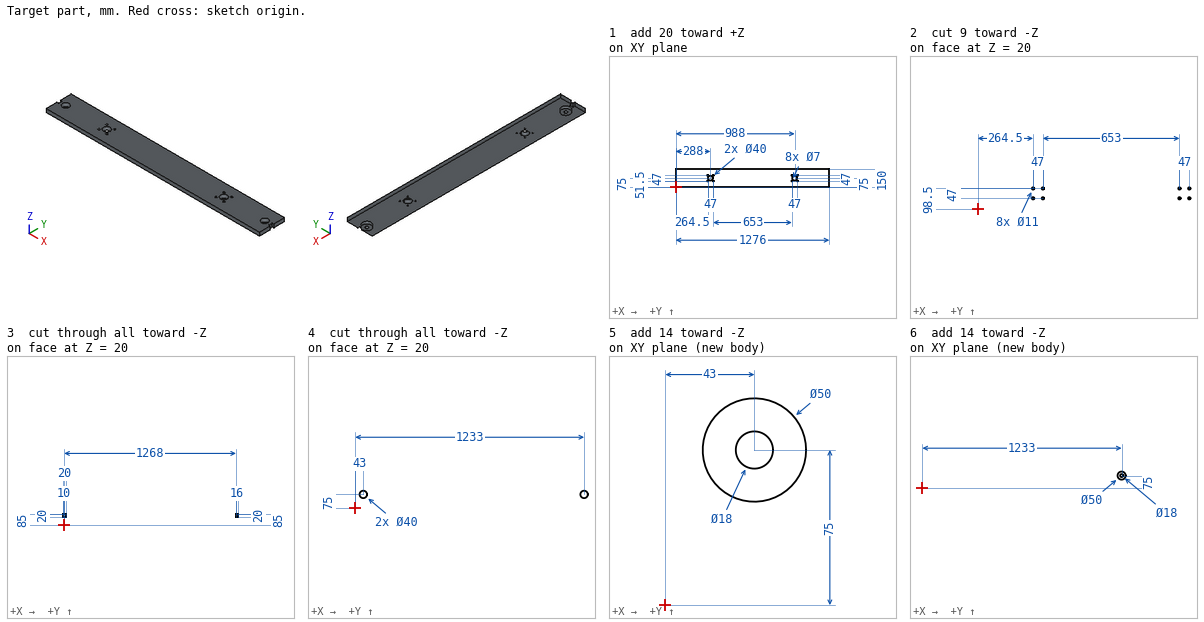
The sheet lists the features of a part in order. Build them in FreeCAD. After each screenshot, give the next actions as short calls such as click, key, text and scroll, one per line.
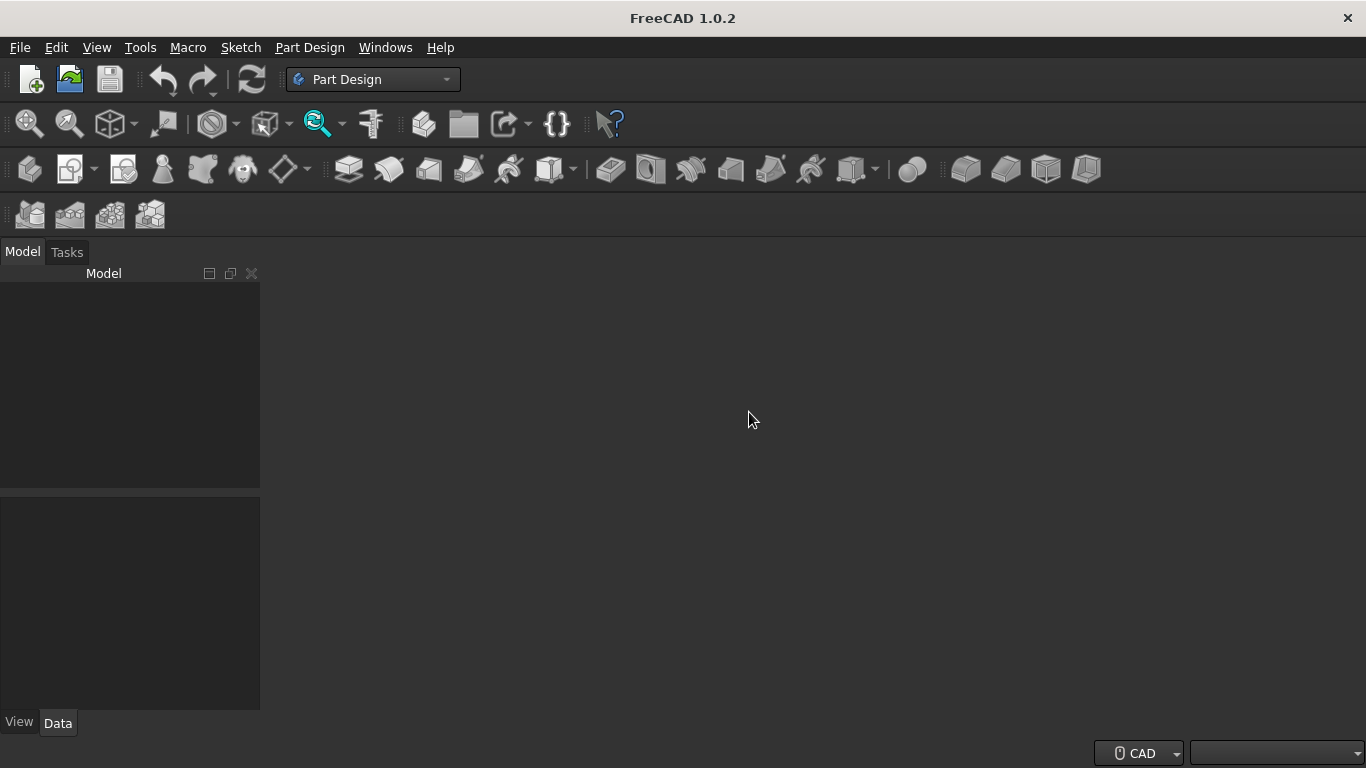
click(30, 80)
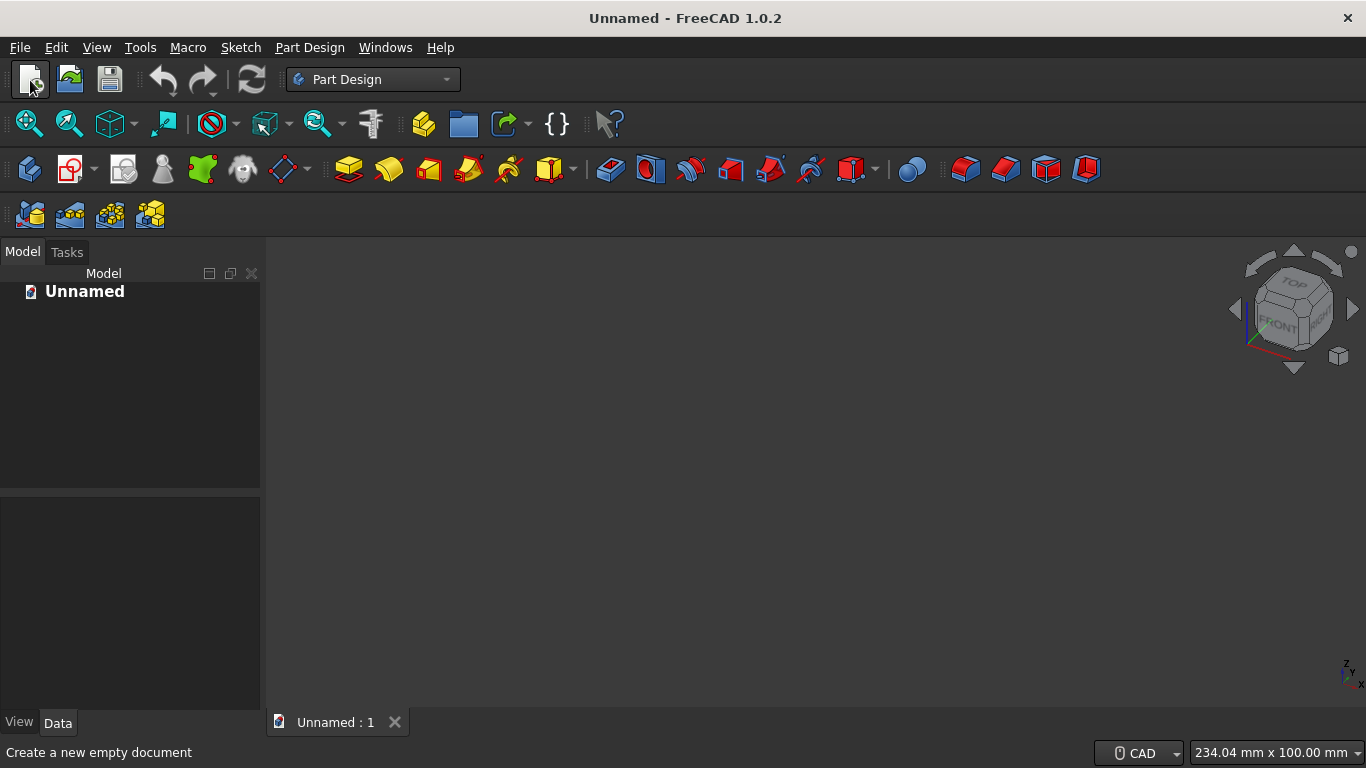
click(70, 170)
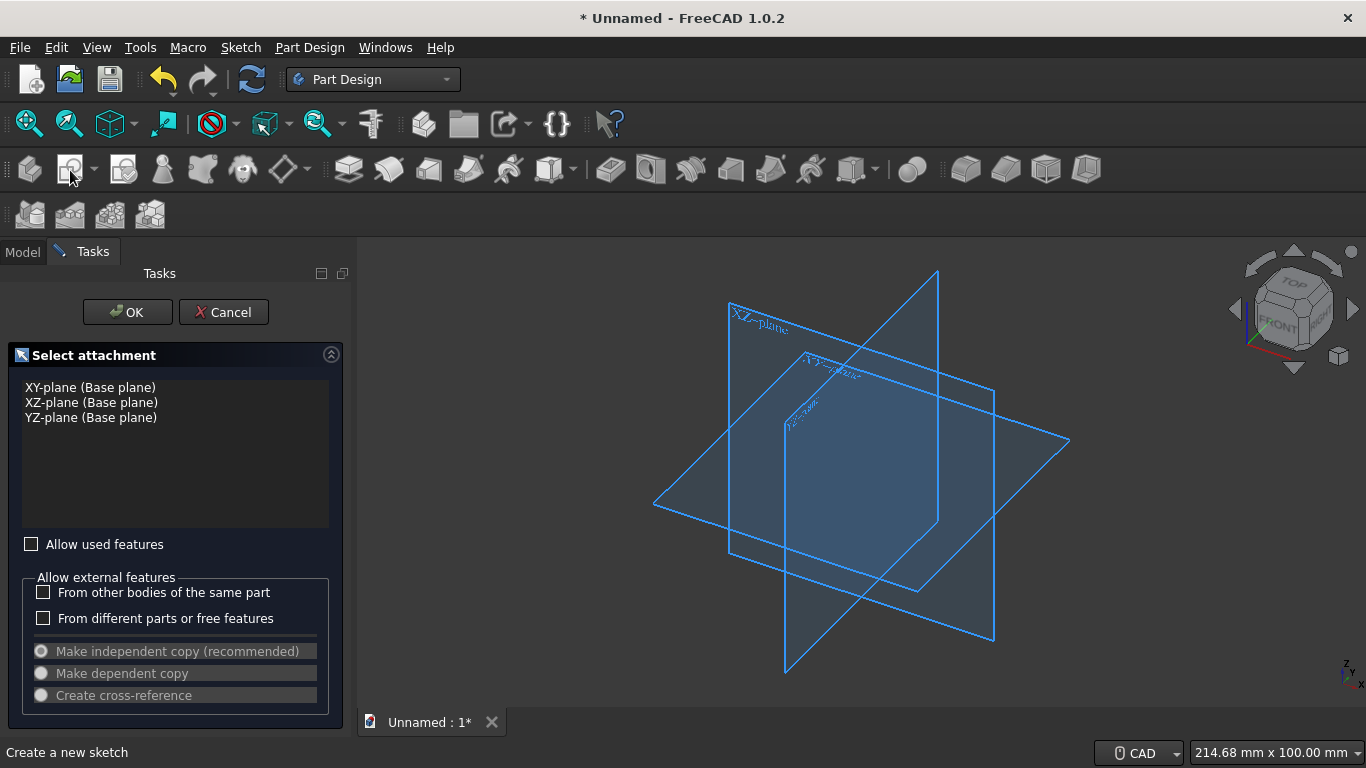
click(82, 388)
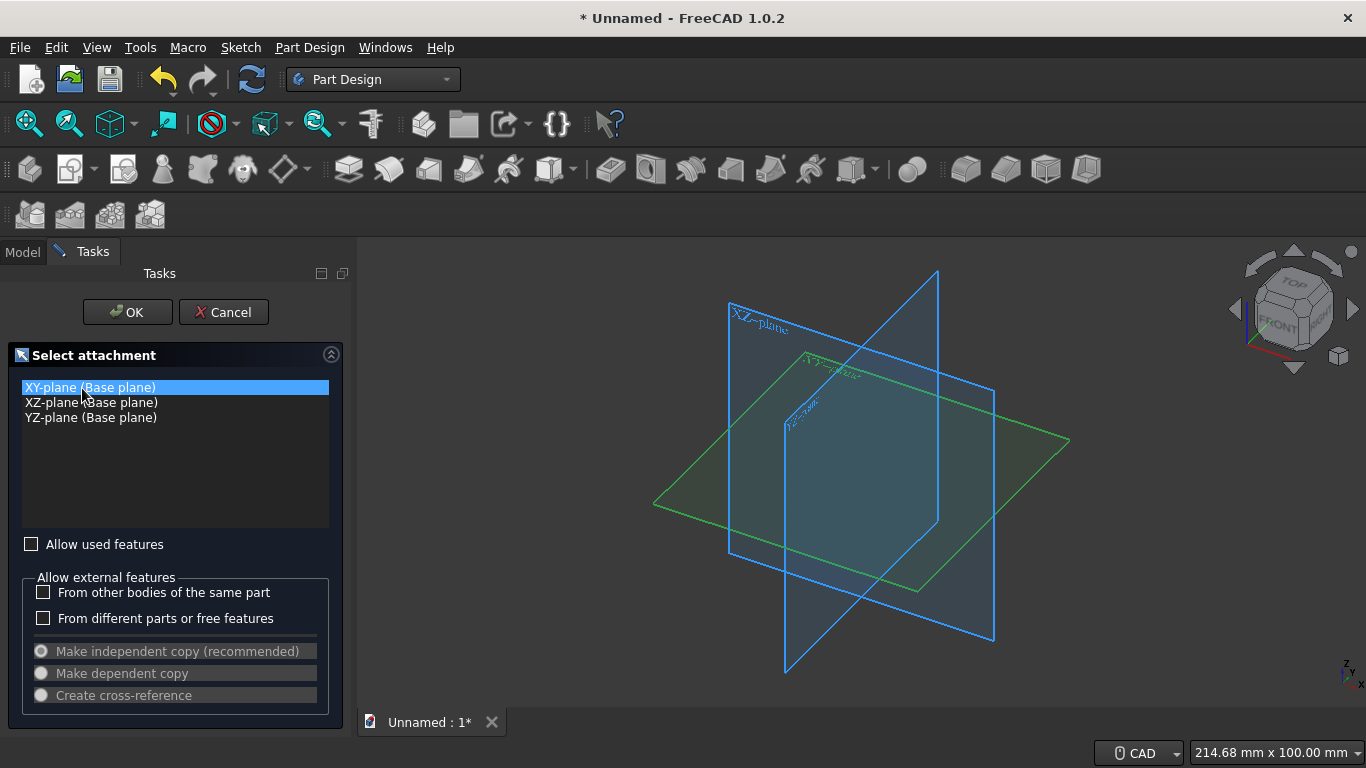
click(128, 312)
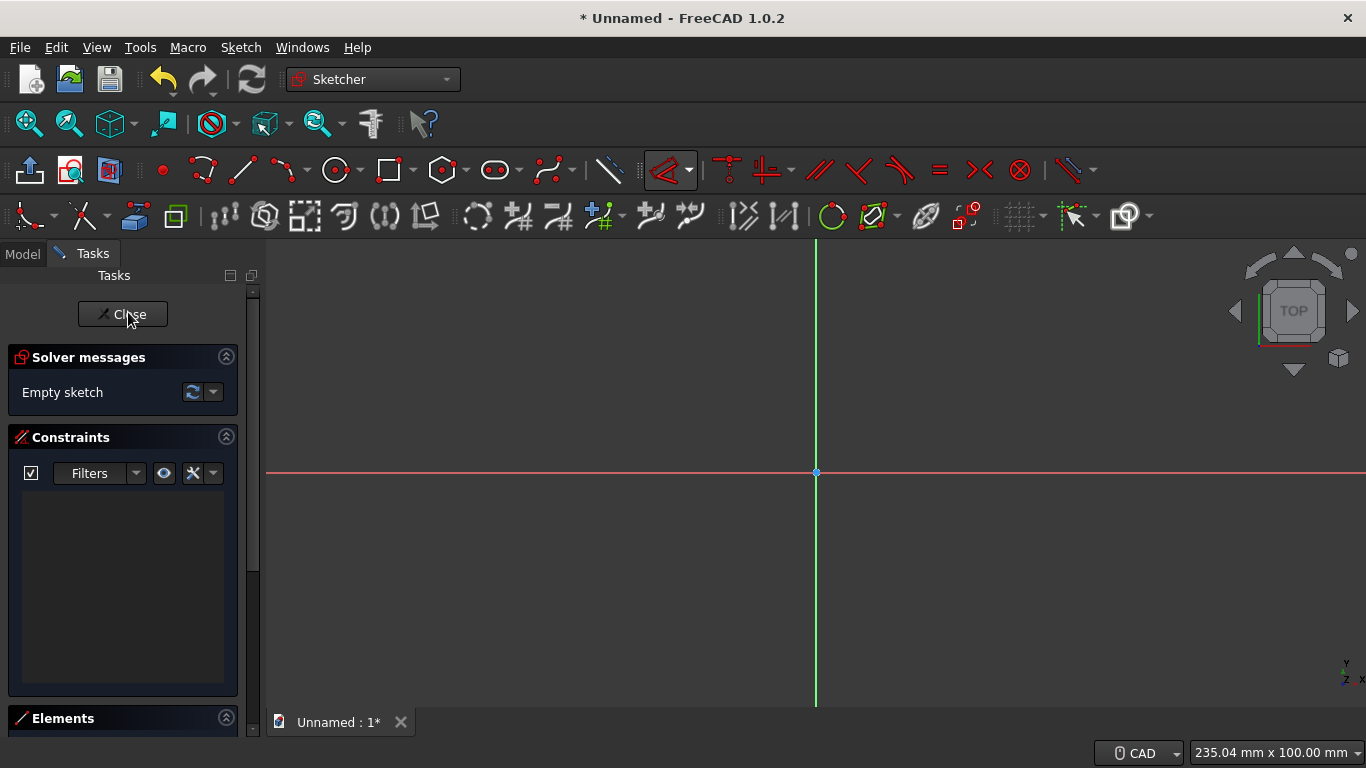
scroll(367, 517, down, 11)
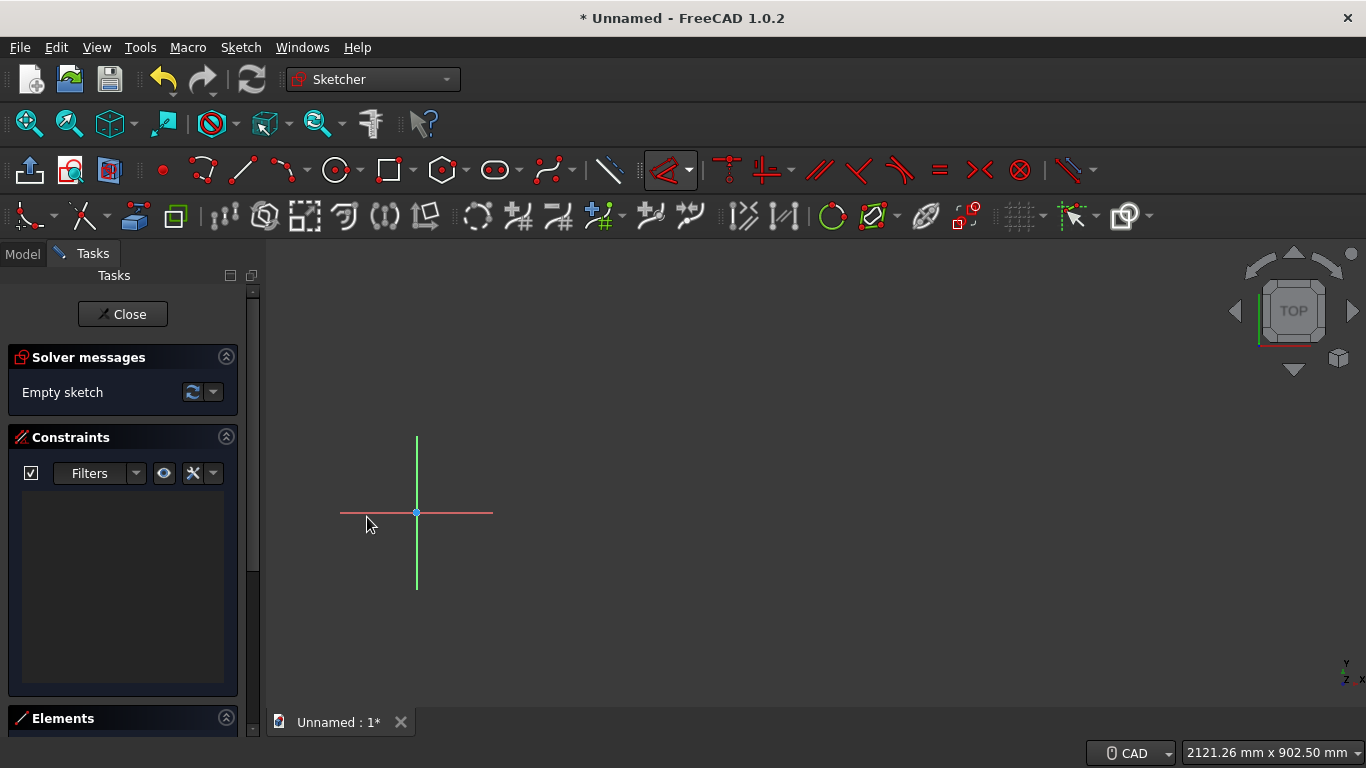
click(390, 170)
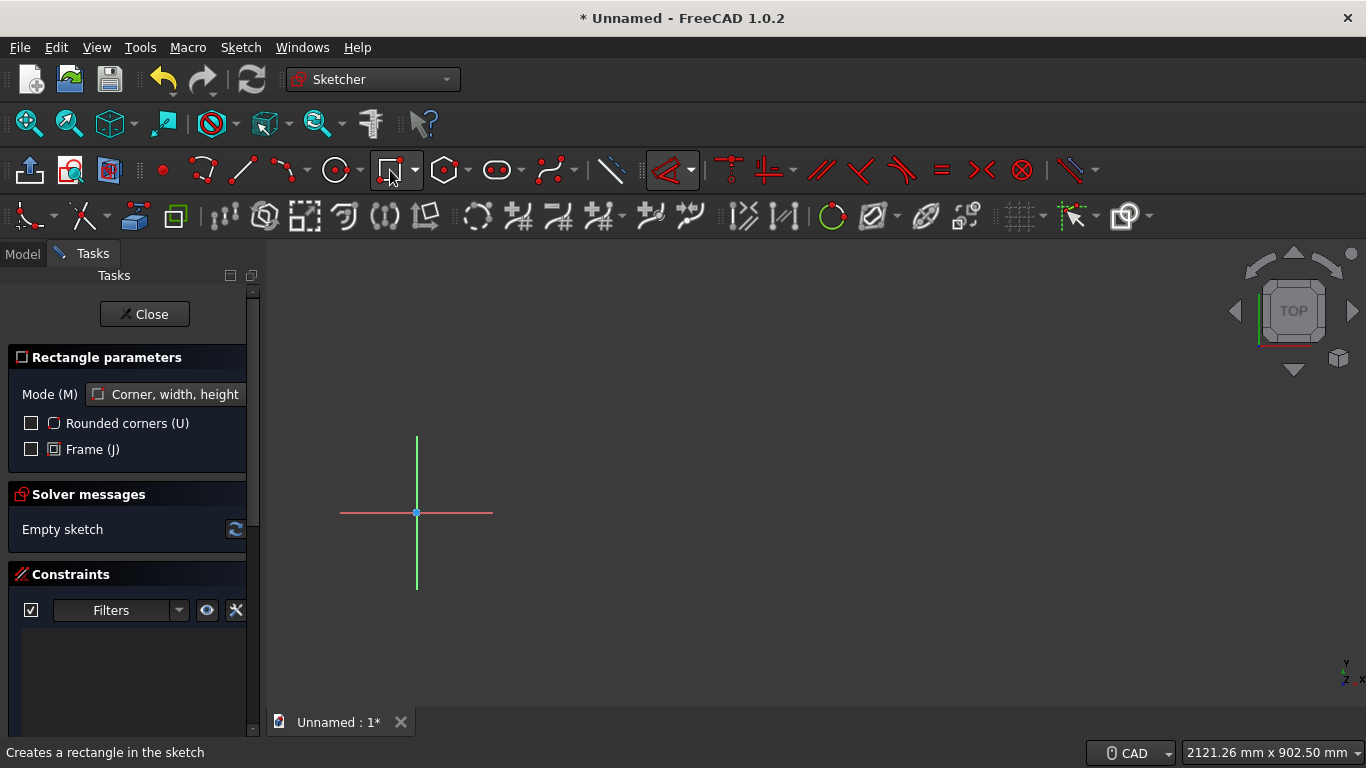
click(417, 513)
move(1079, 435)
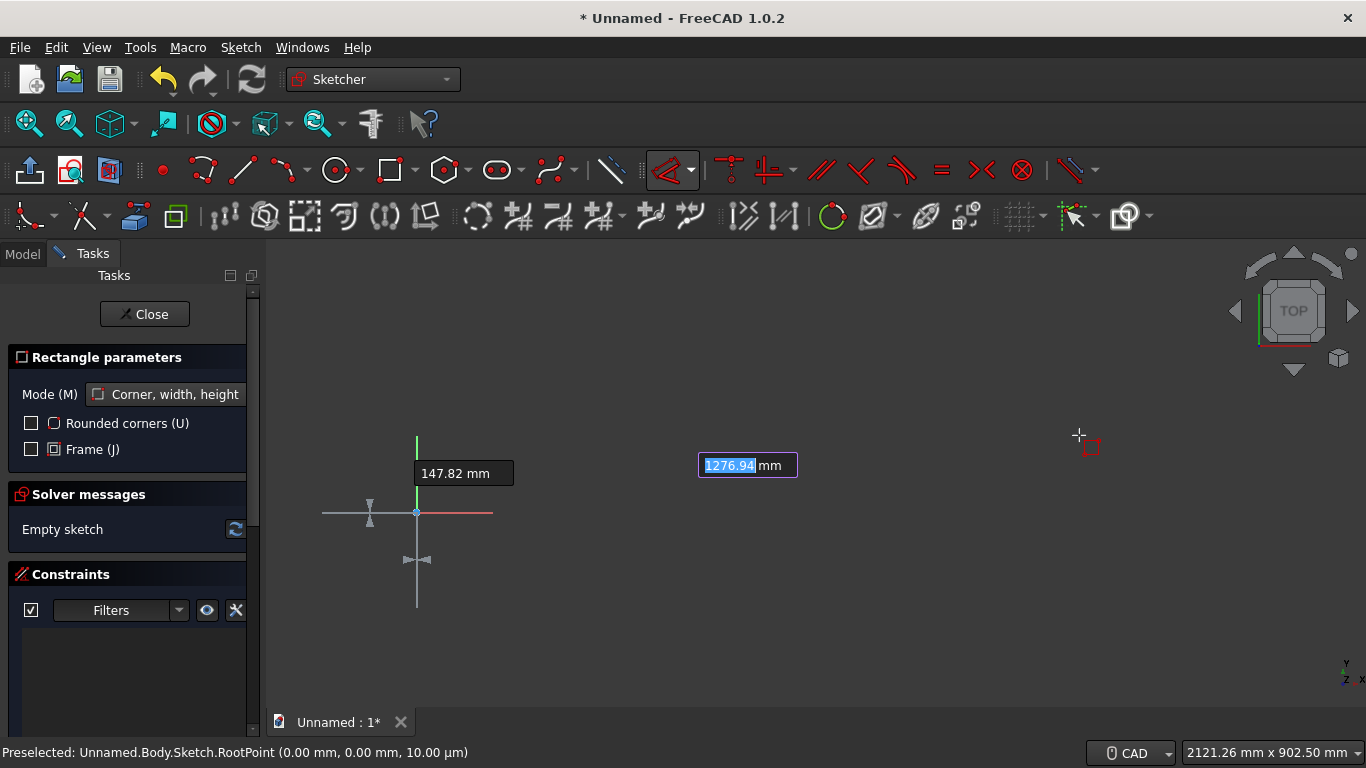
text(1276)
key(Tab)
text(150)
key(Return)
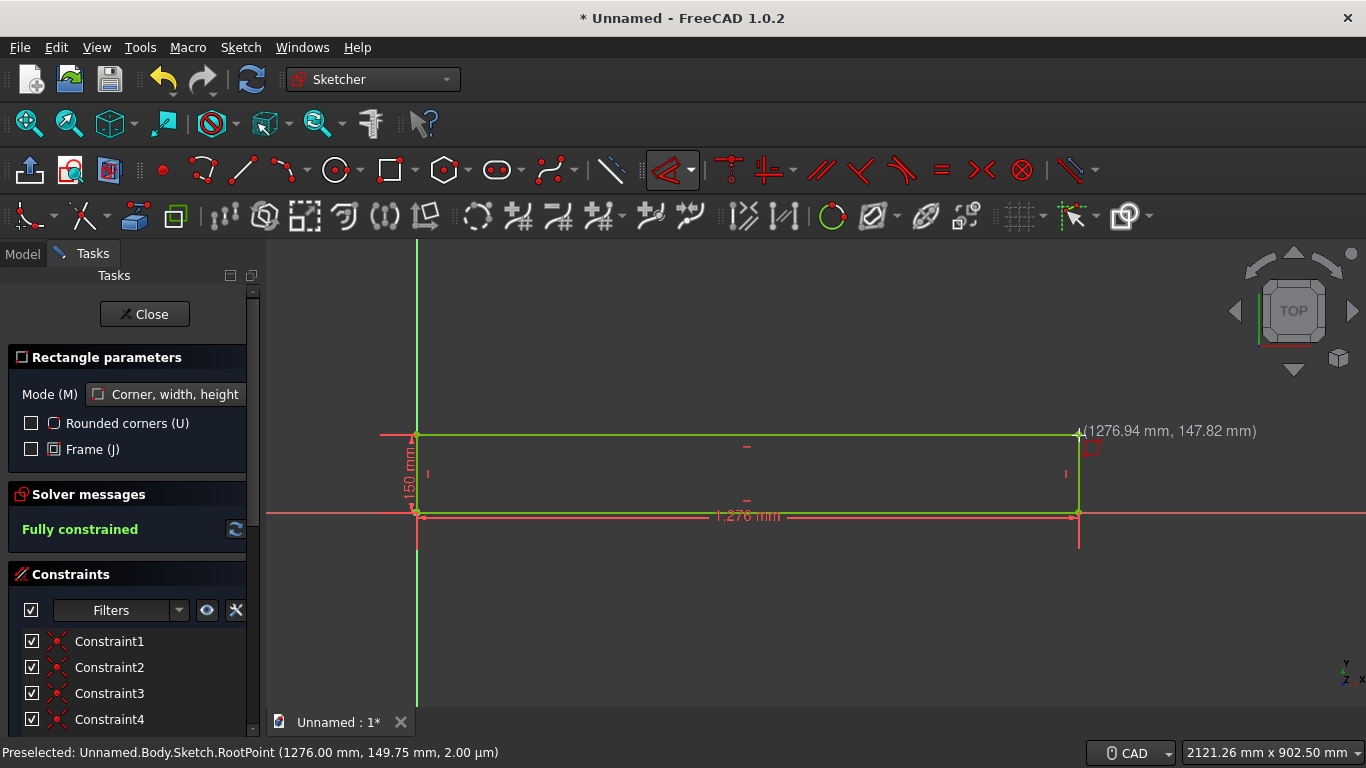
click(336, 170)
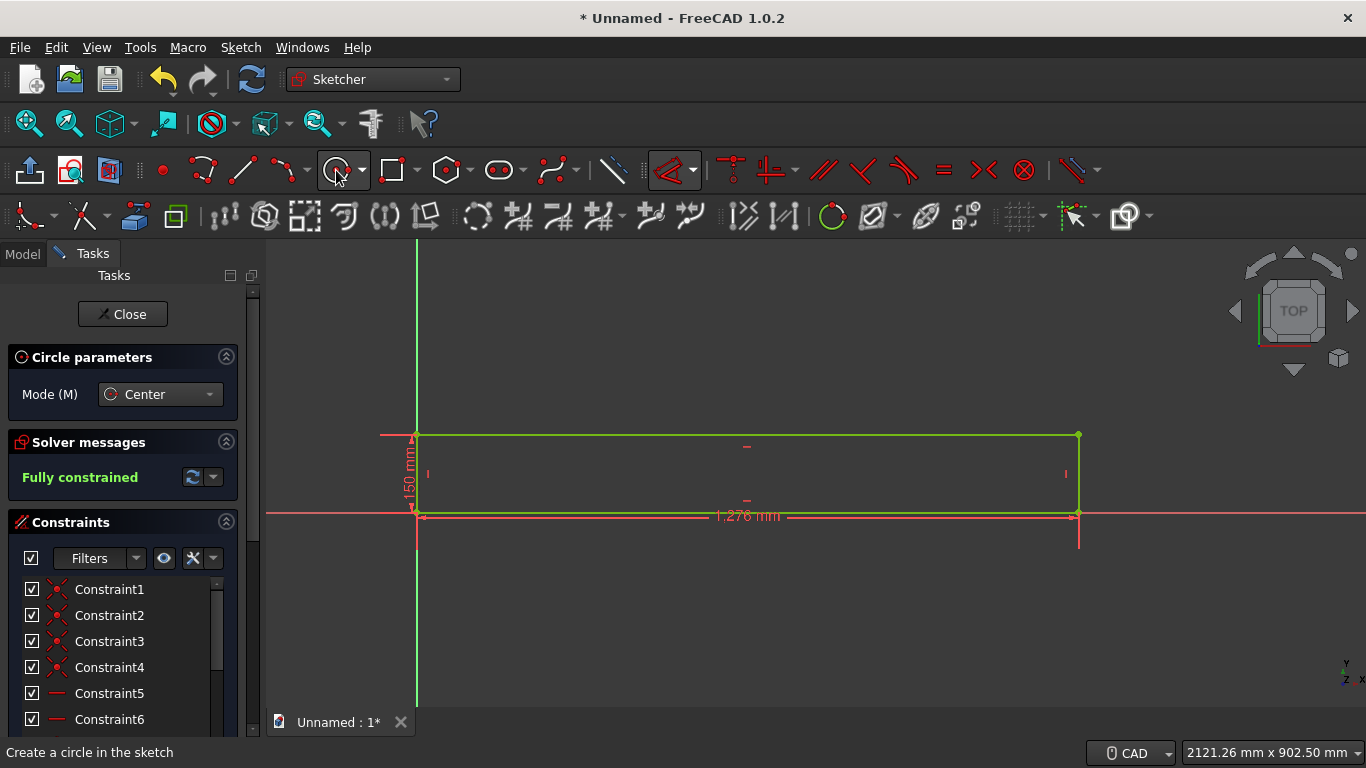
scroll(554, 486, up, 13)